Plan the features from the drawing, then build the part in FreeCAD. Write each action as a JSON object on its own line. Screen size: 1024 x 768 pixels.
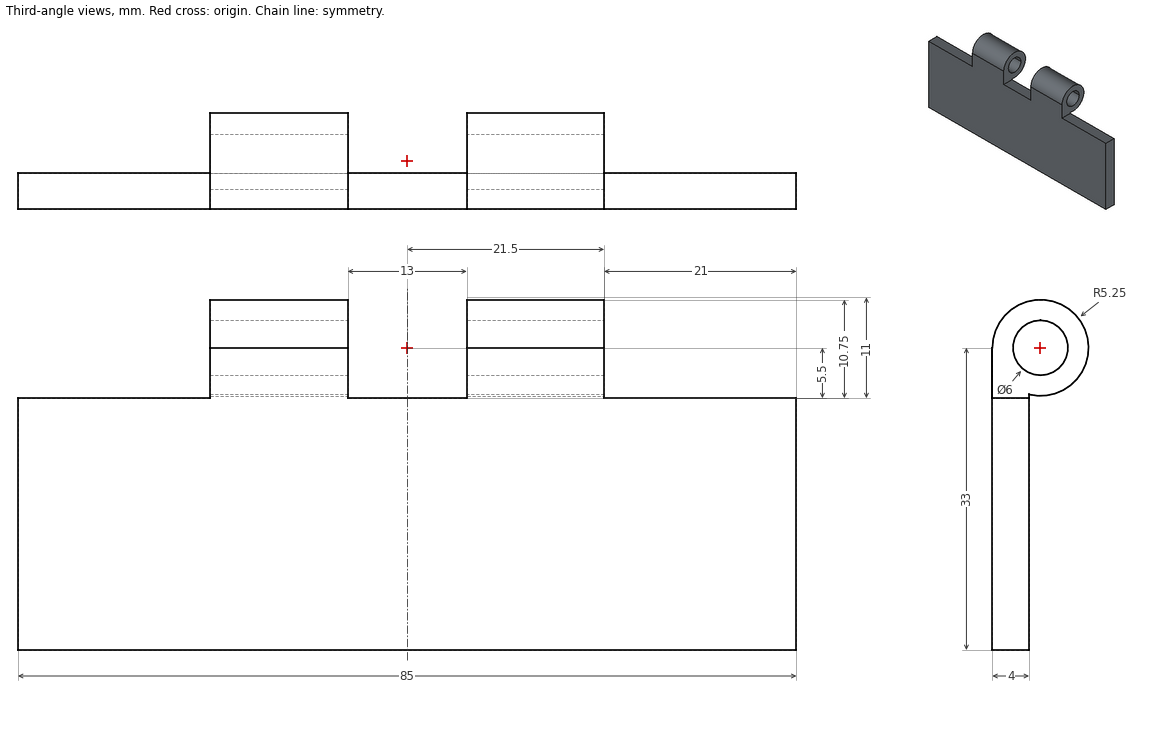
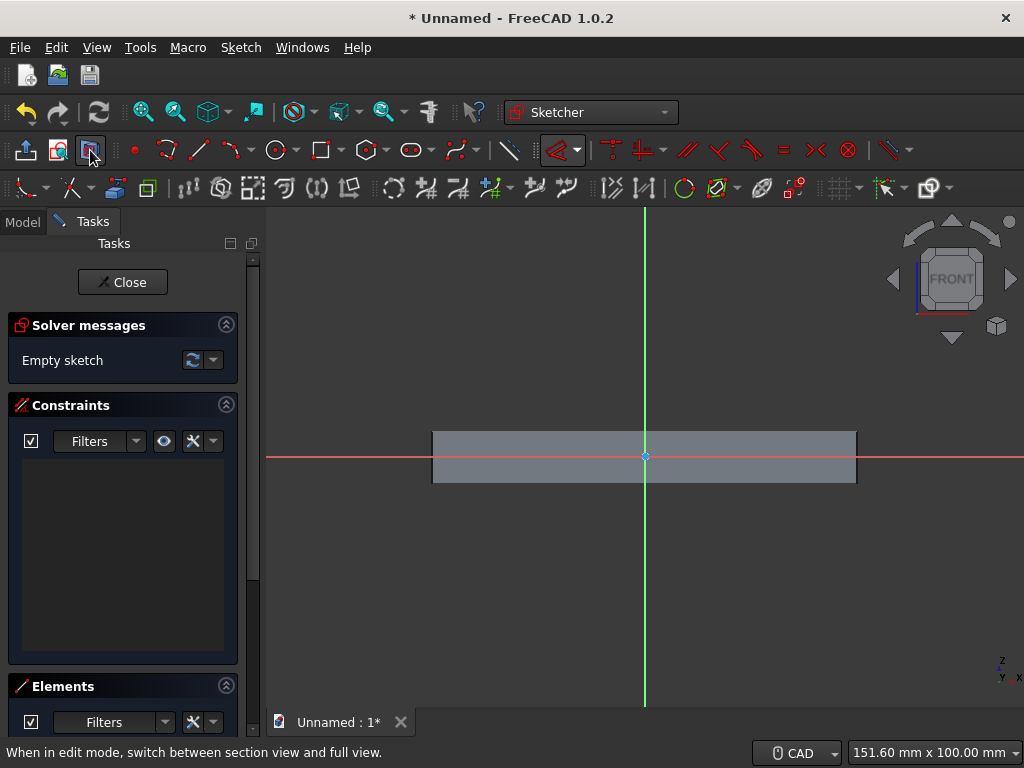
{"action": "scroll", "coordinate": [294, 457], "scroll_direction": "down", "scroll_amount": 1}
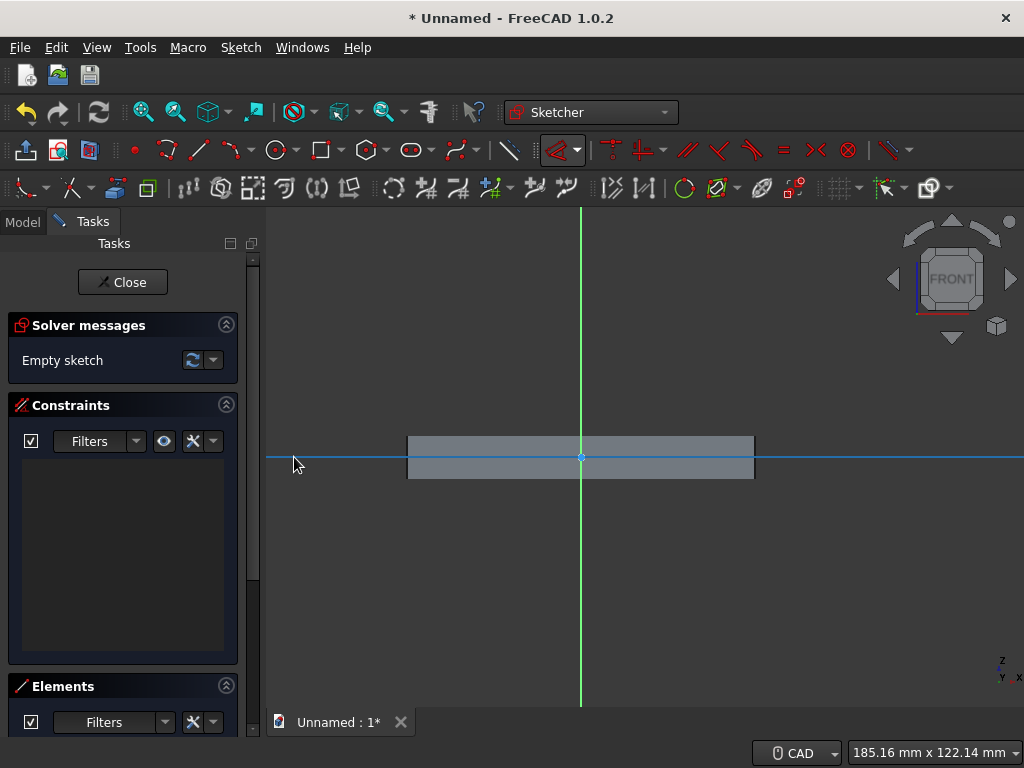
{"action": "left_click", "coordinate": [344, 150]}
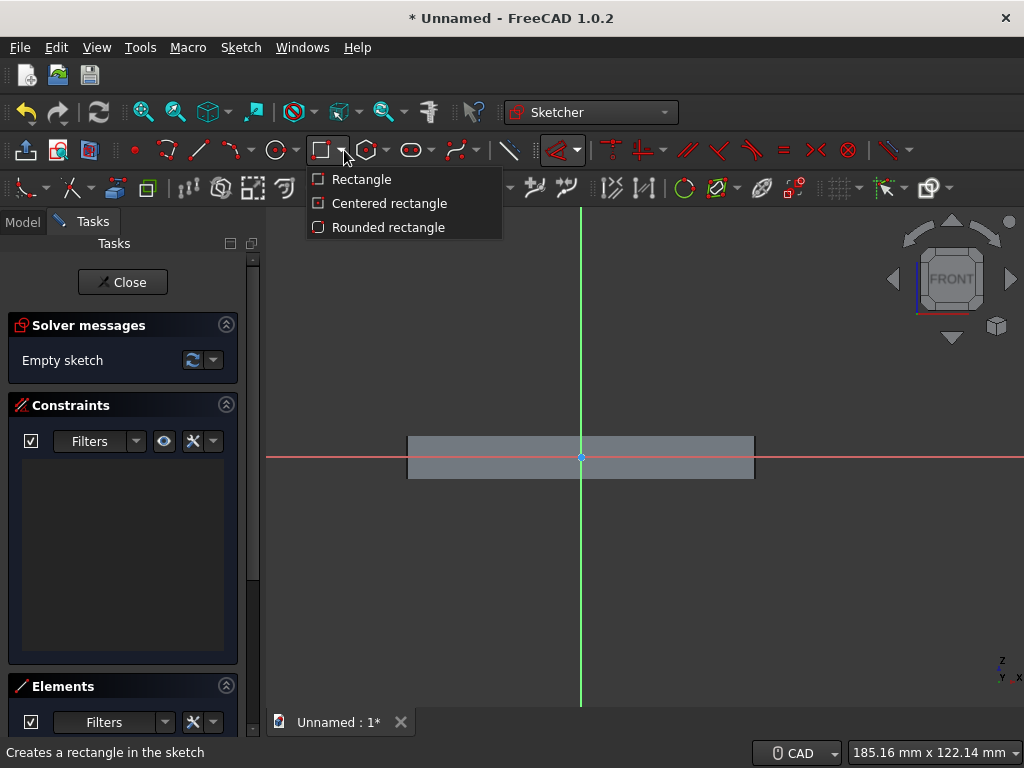
{"action": "left_click", "coordinate": [404, 203]}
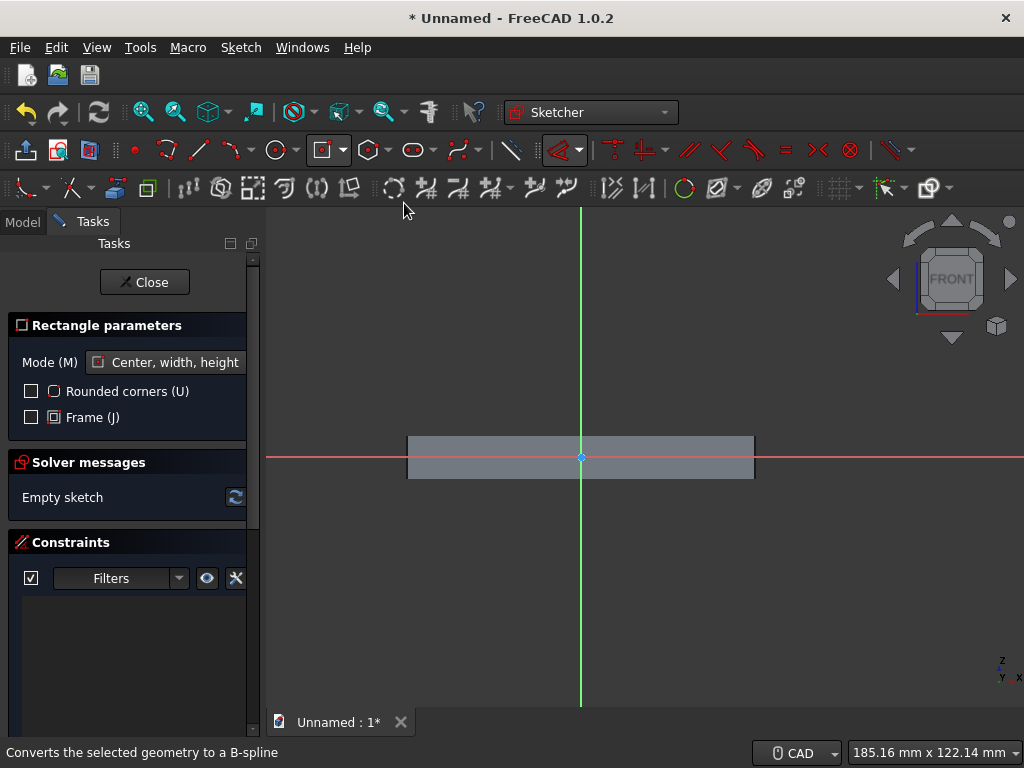
{"action": "left_click", "coordinate": [581, 457]}
{"action": "left_click", "coordinate": [608, 435]}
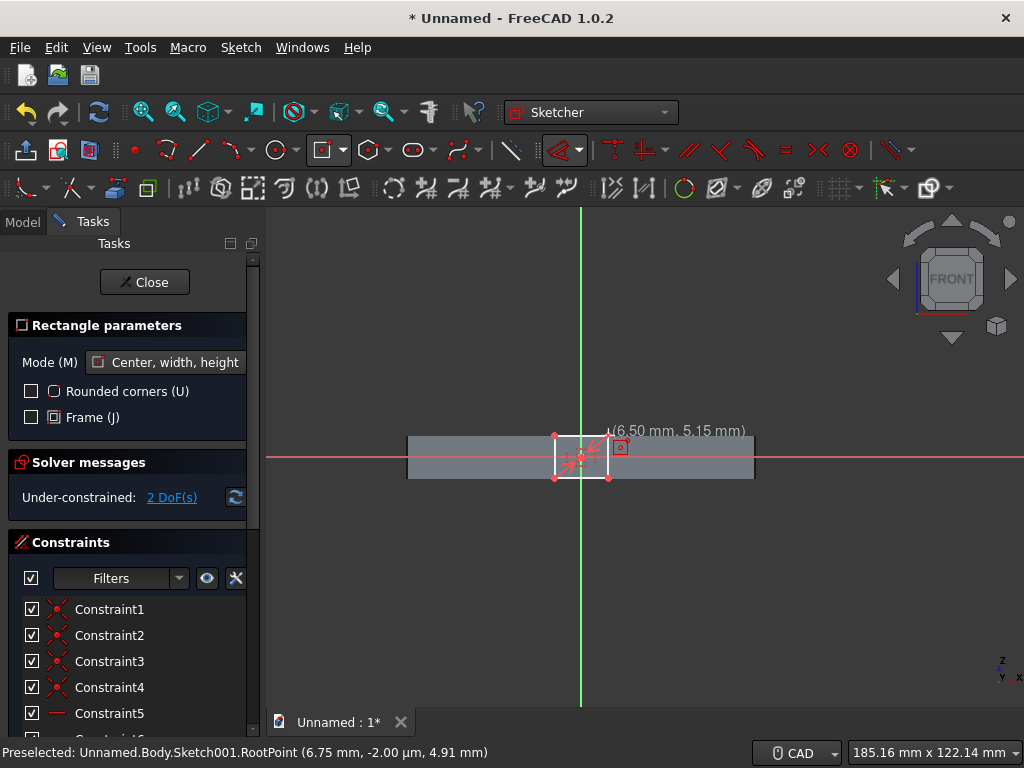
{"action": "left_click", "coordinate": [346, 150]}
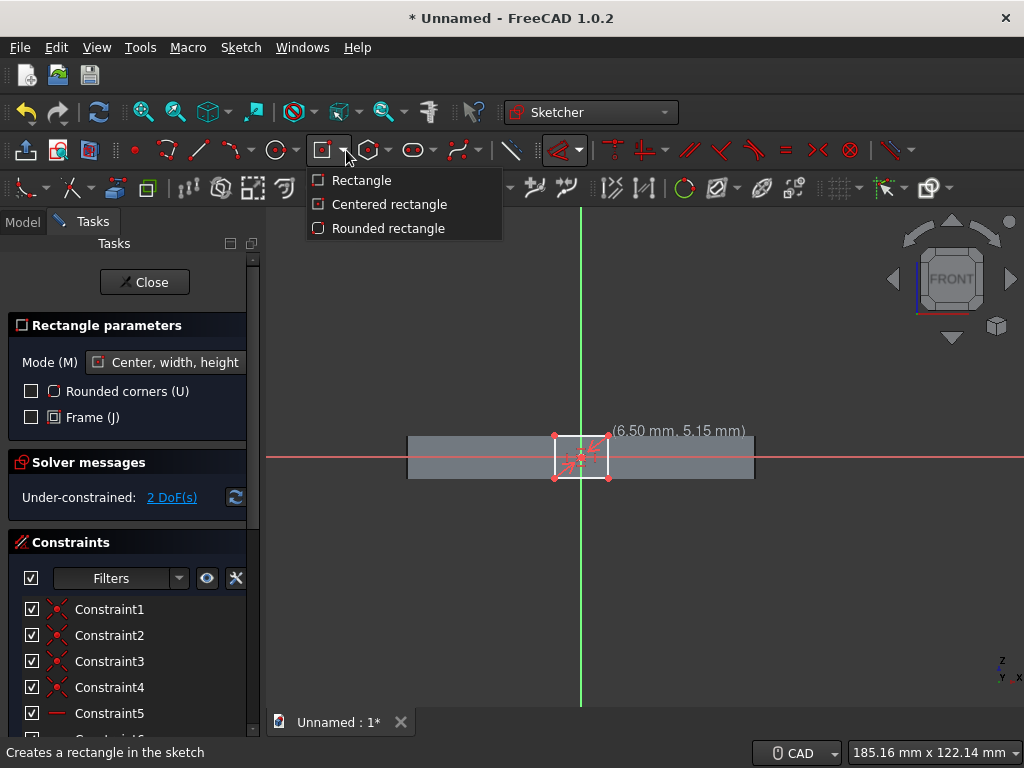
{"action": "left_click", "coordinate": [404, 180]}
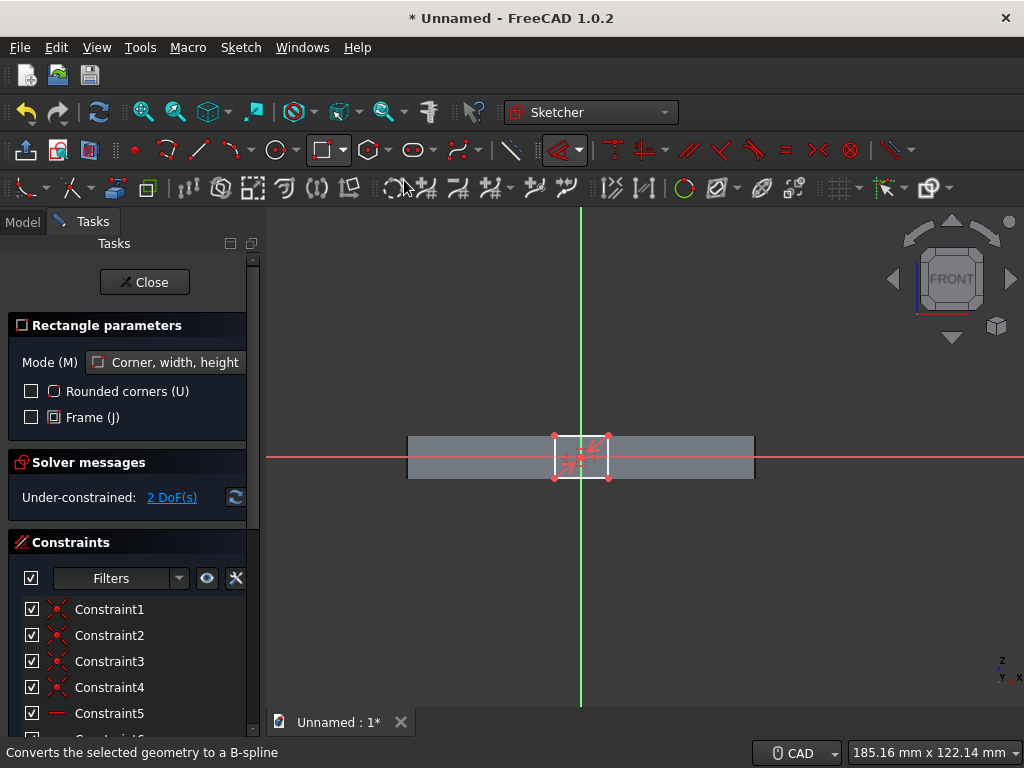
{"action": "left_click", "coordinate": [669, 436]}
{"action": "left_click", "coordinate": [755, 480]}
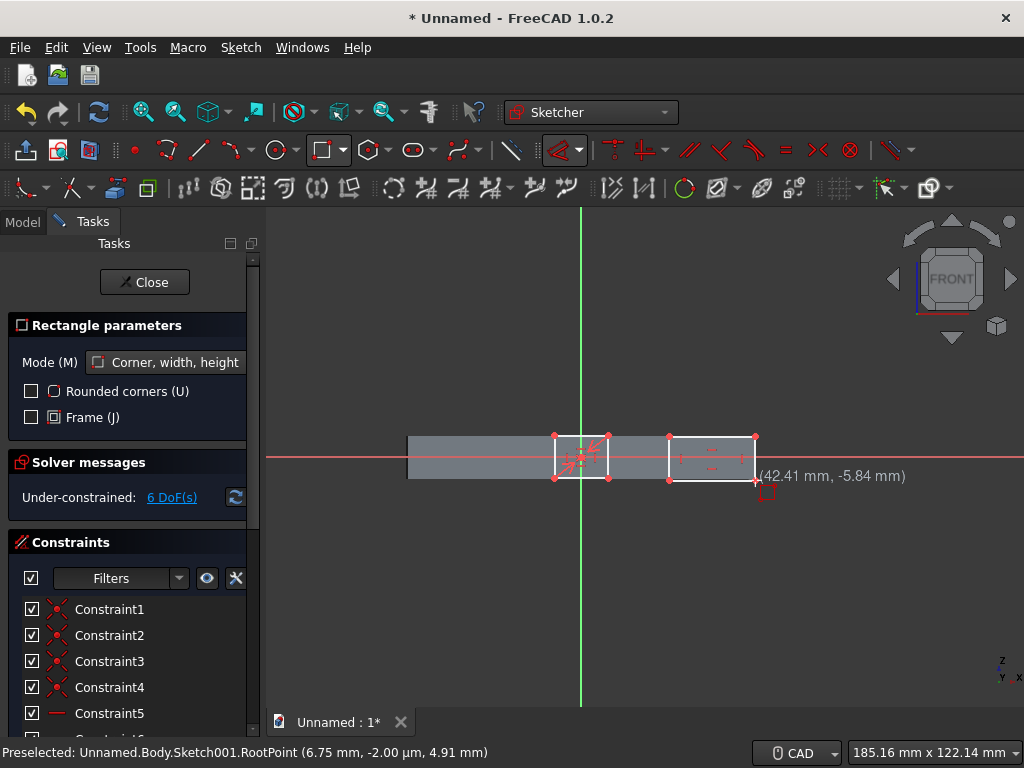
{"action": "left_click", "coordinate": [407, 436]}
{"action": "left_click", "coordinate": [493, 480]}
{"action": "key", "text": "Escape"}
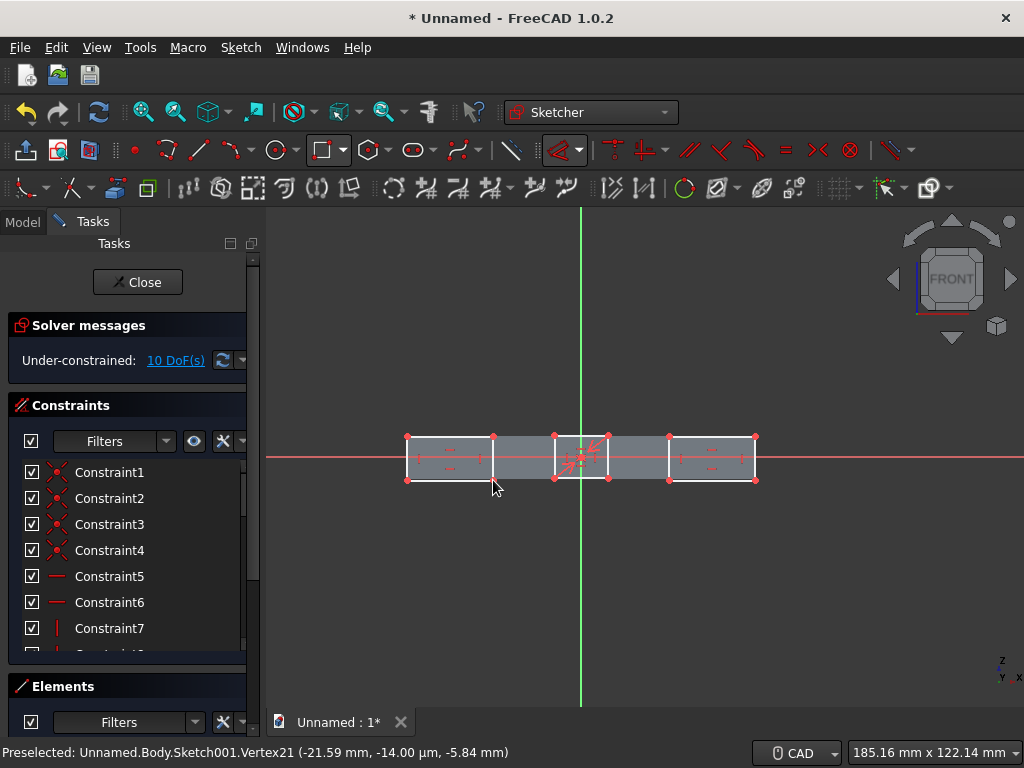
{"action": "left_click", "coordinate": [755, 437]}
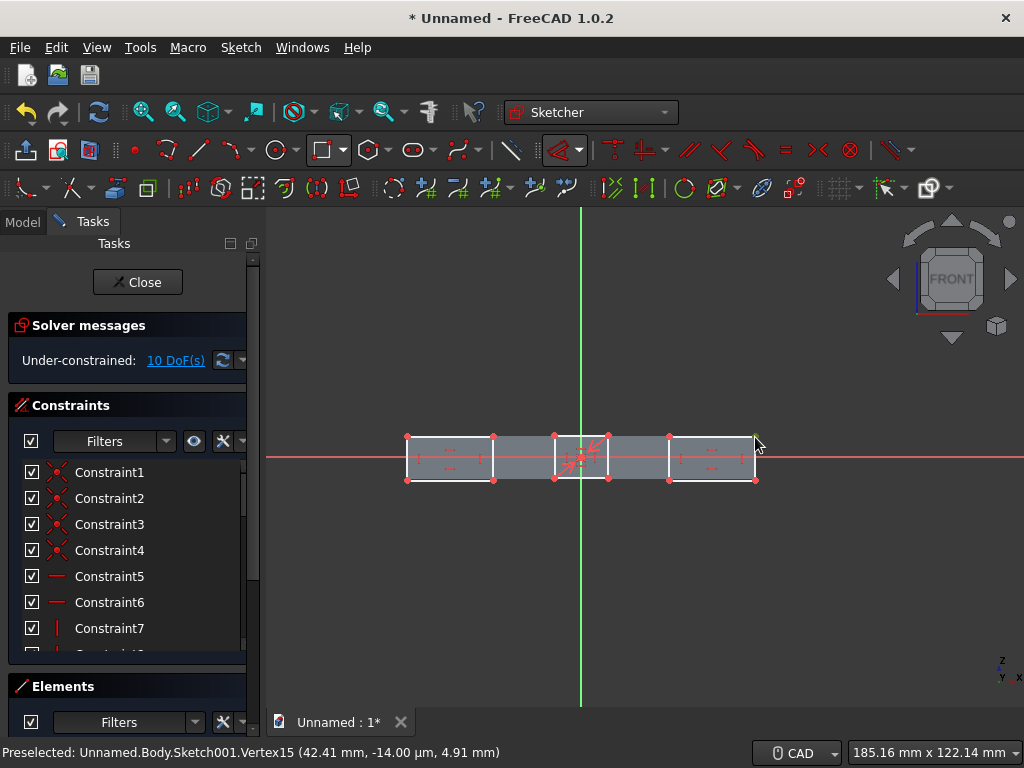
{"action": "left_click", "coordinate": [407, 437]}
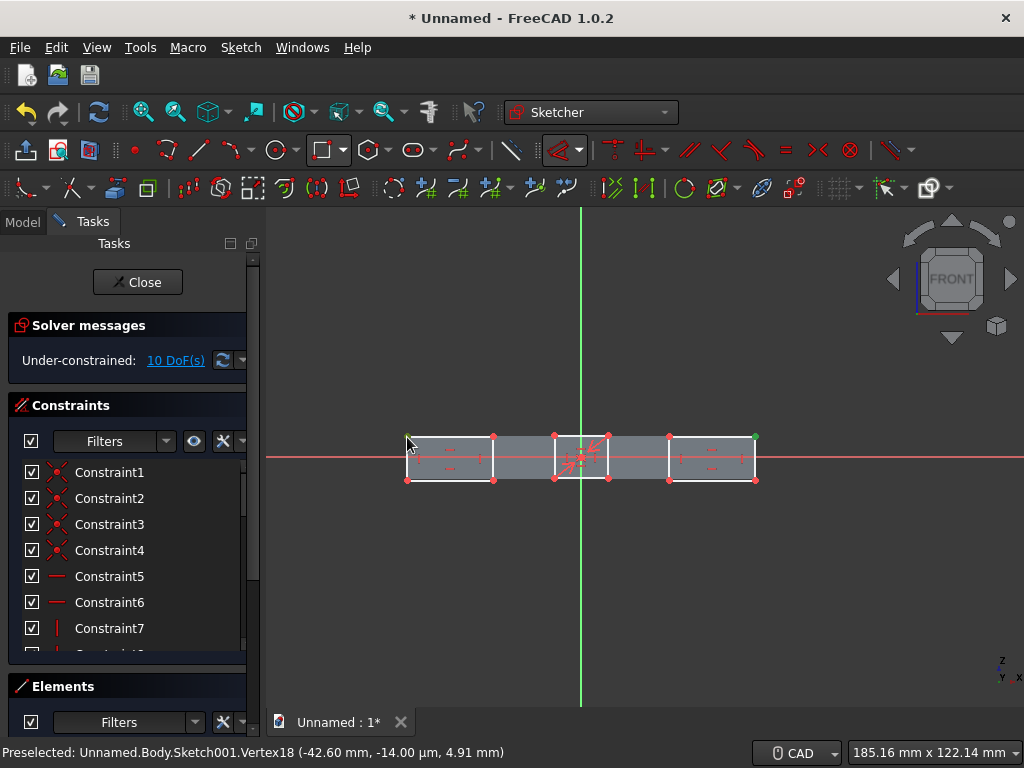
{"action": "left_click", "coordinate": [581, 647]}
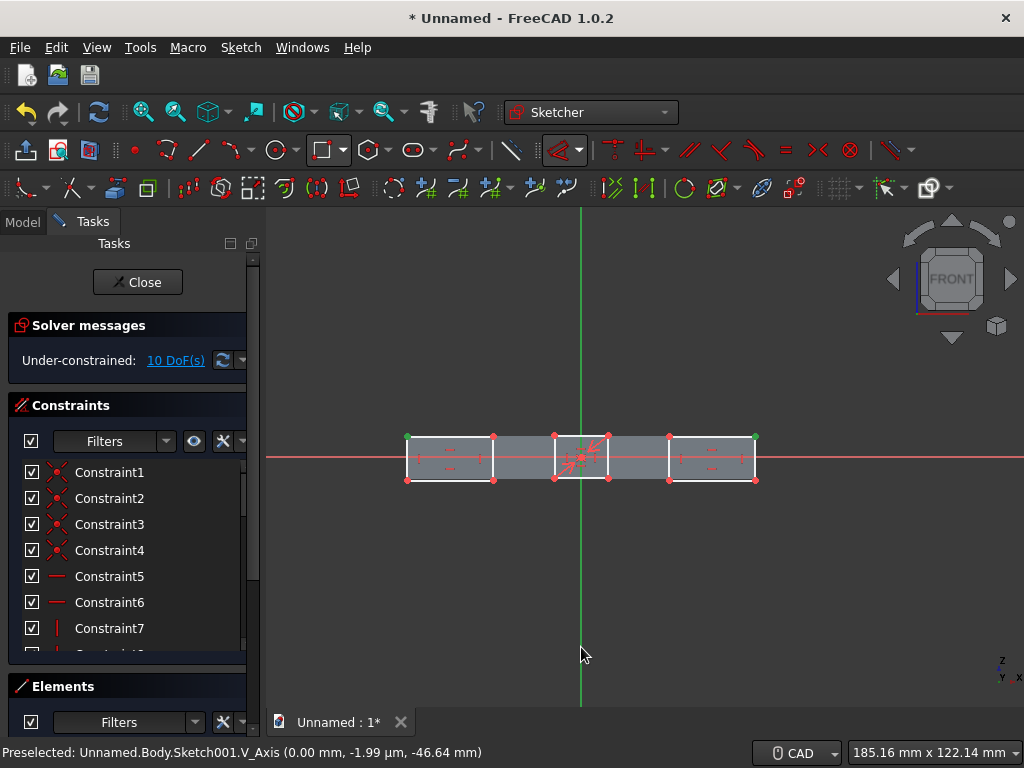
{"action": "left_click", "coordinate": [818, 150]}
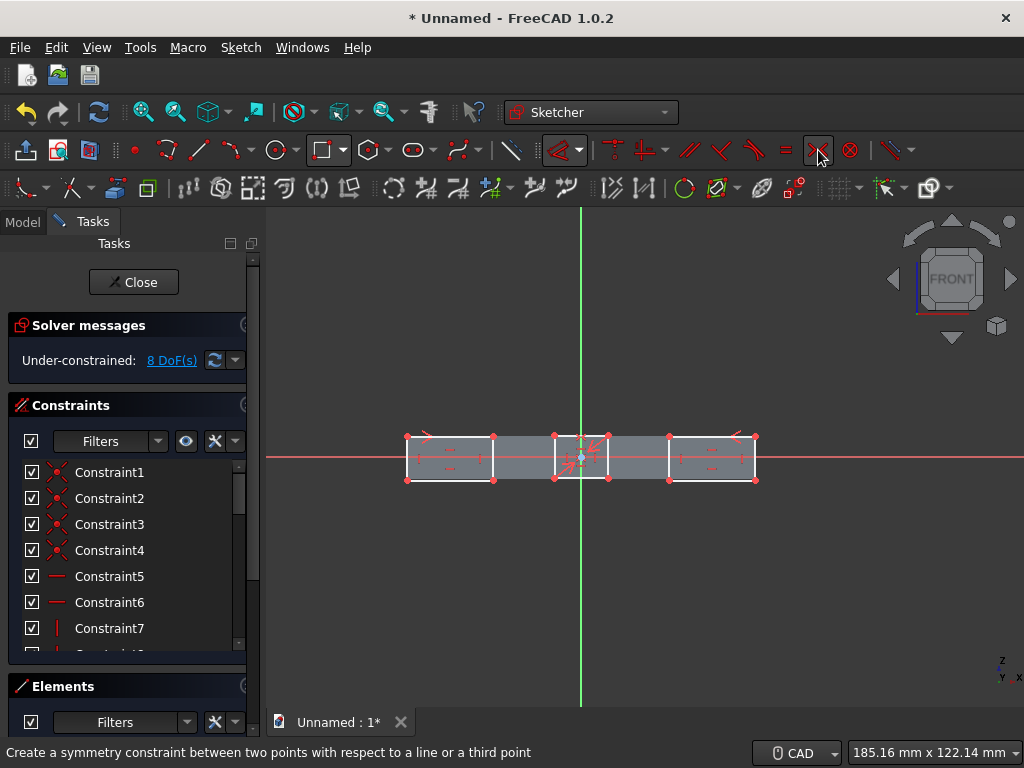
{"action": "left_click", "coordinate": [669, 481]}